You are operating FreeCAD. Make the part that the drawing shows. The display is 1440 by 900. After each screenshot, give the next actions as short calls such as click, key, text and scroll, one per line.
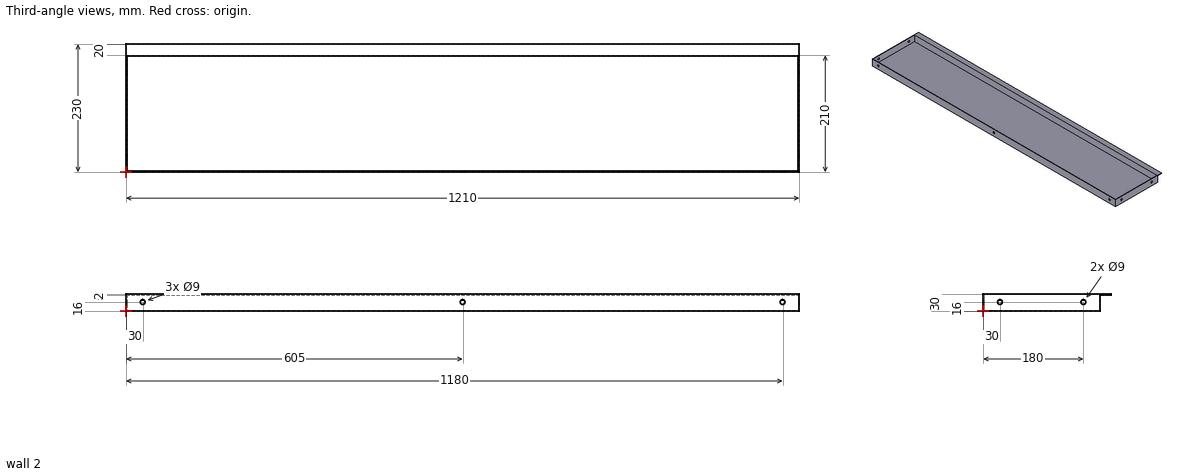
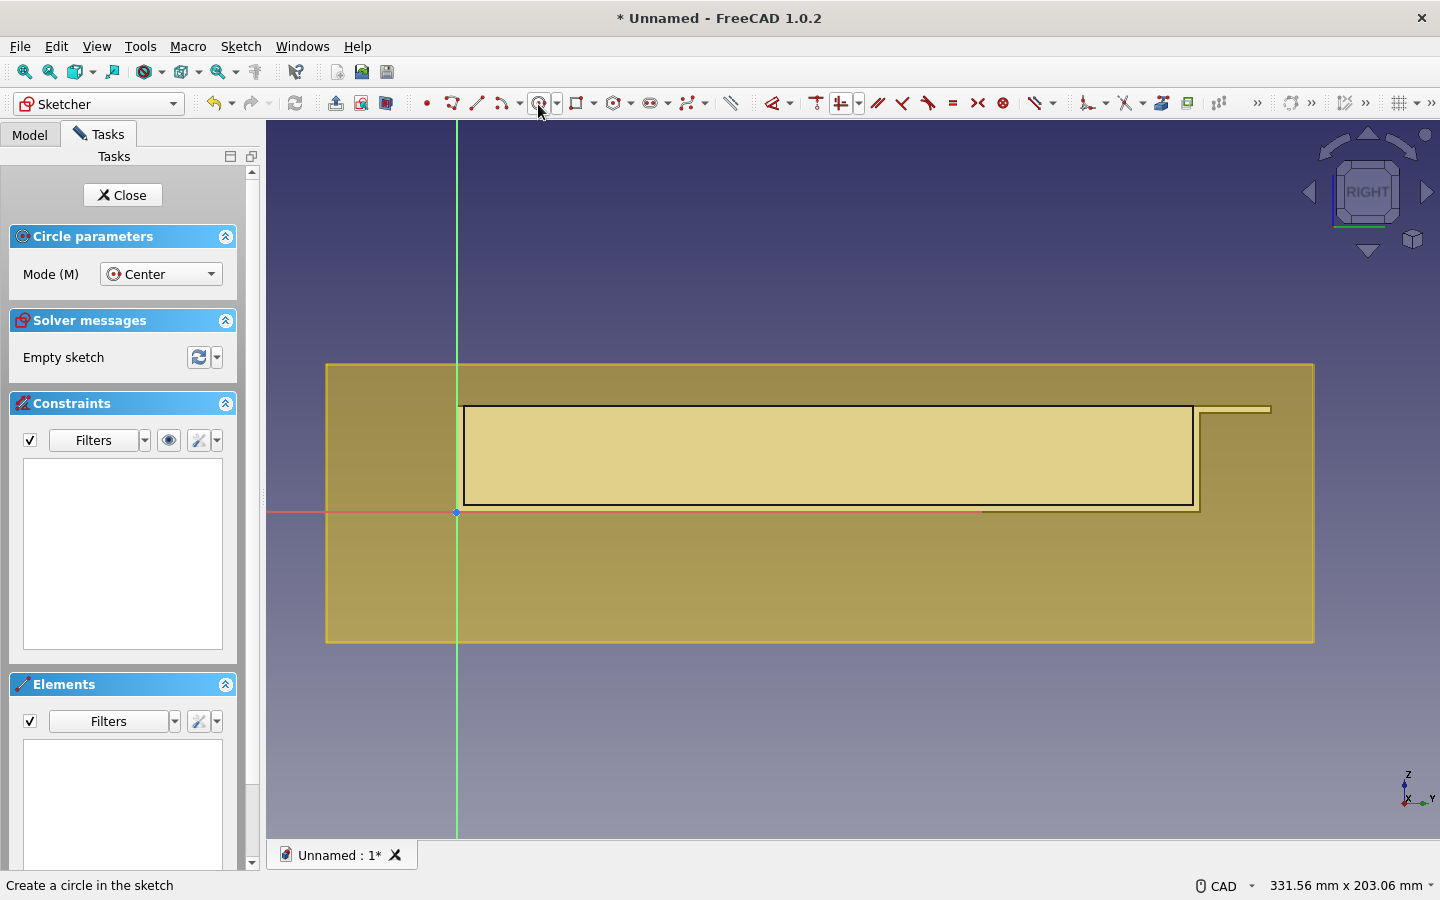
scroll(1094, 456, up, 2)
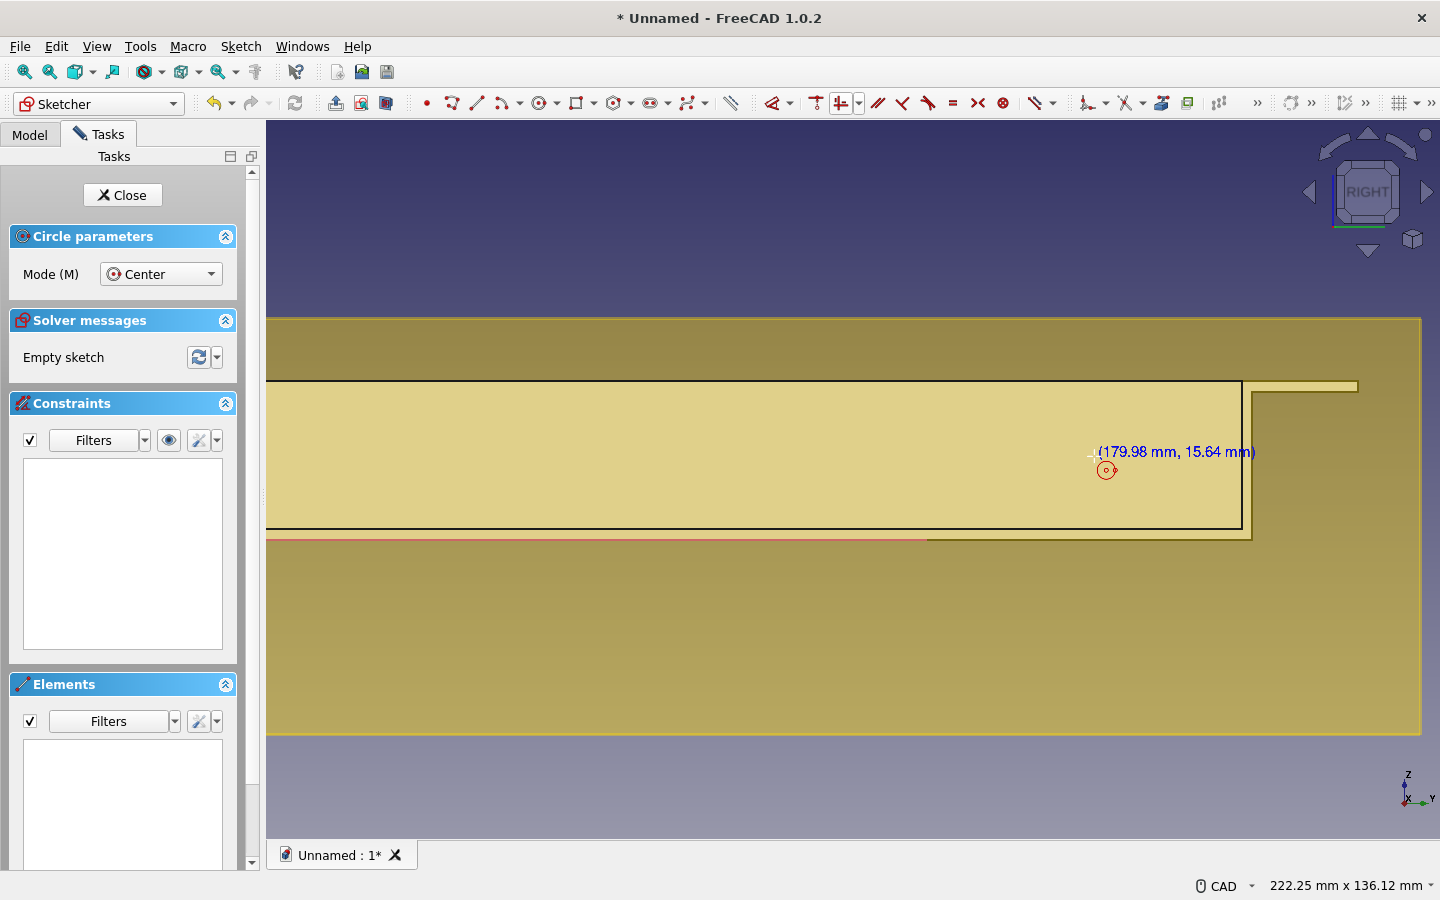
click(1094, 455)
click(1111, 439)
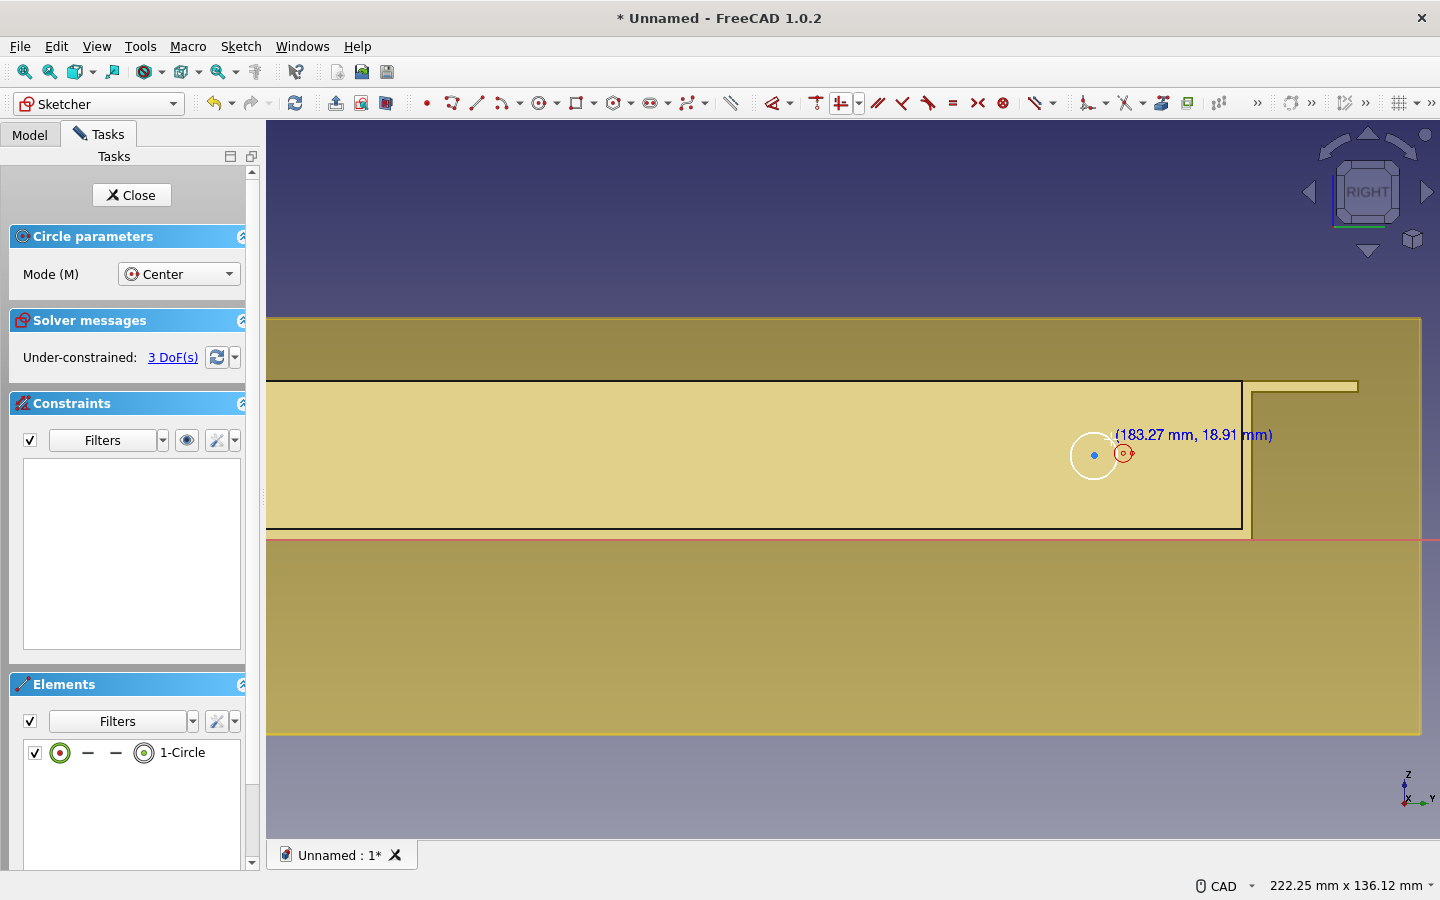
click(301, 455)
click(318, 439)
key(Escape)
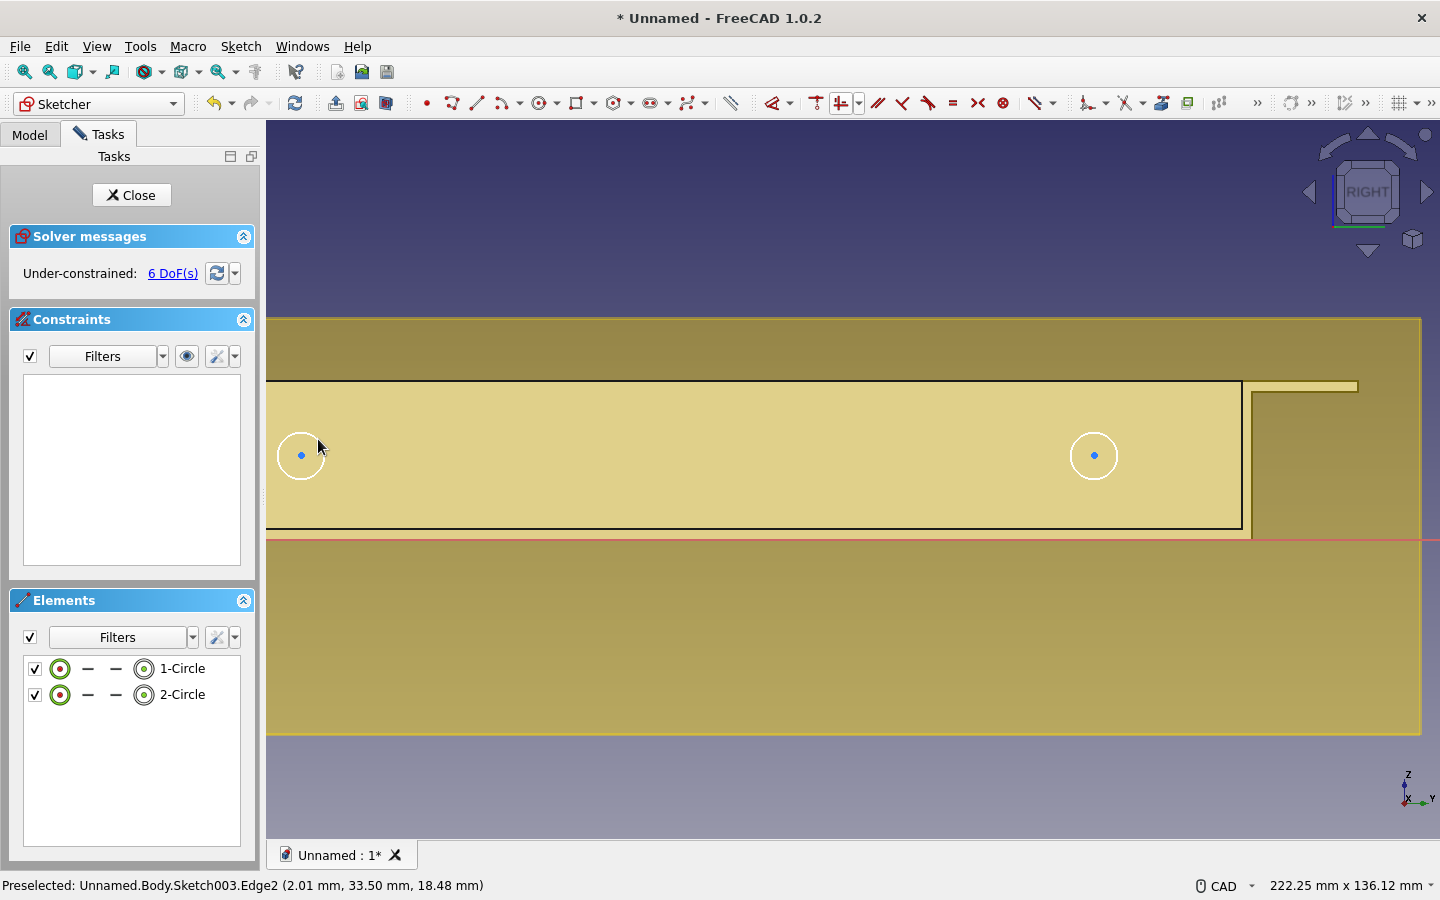
click(1110, 439)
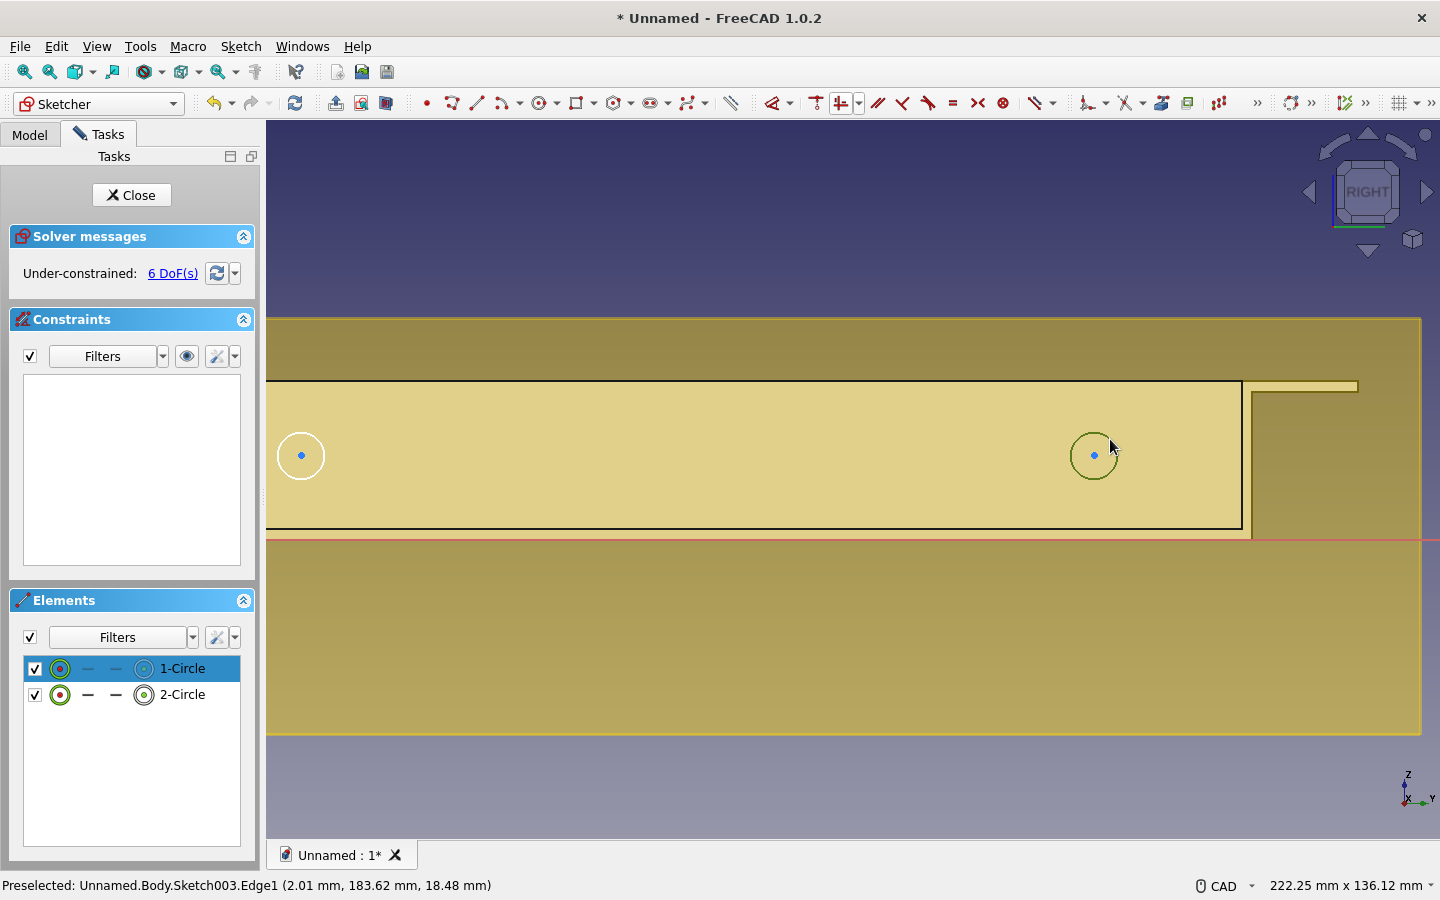
click(317, 439)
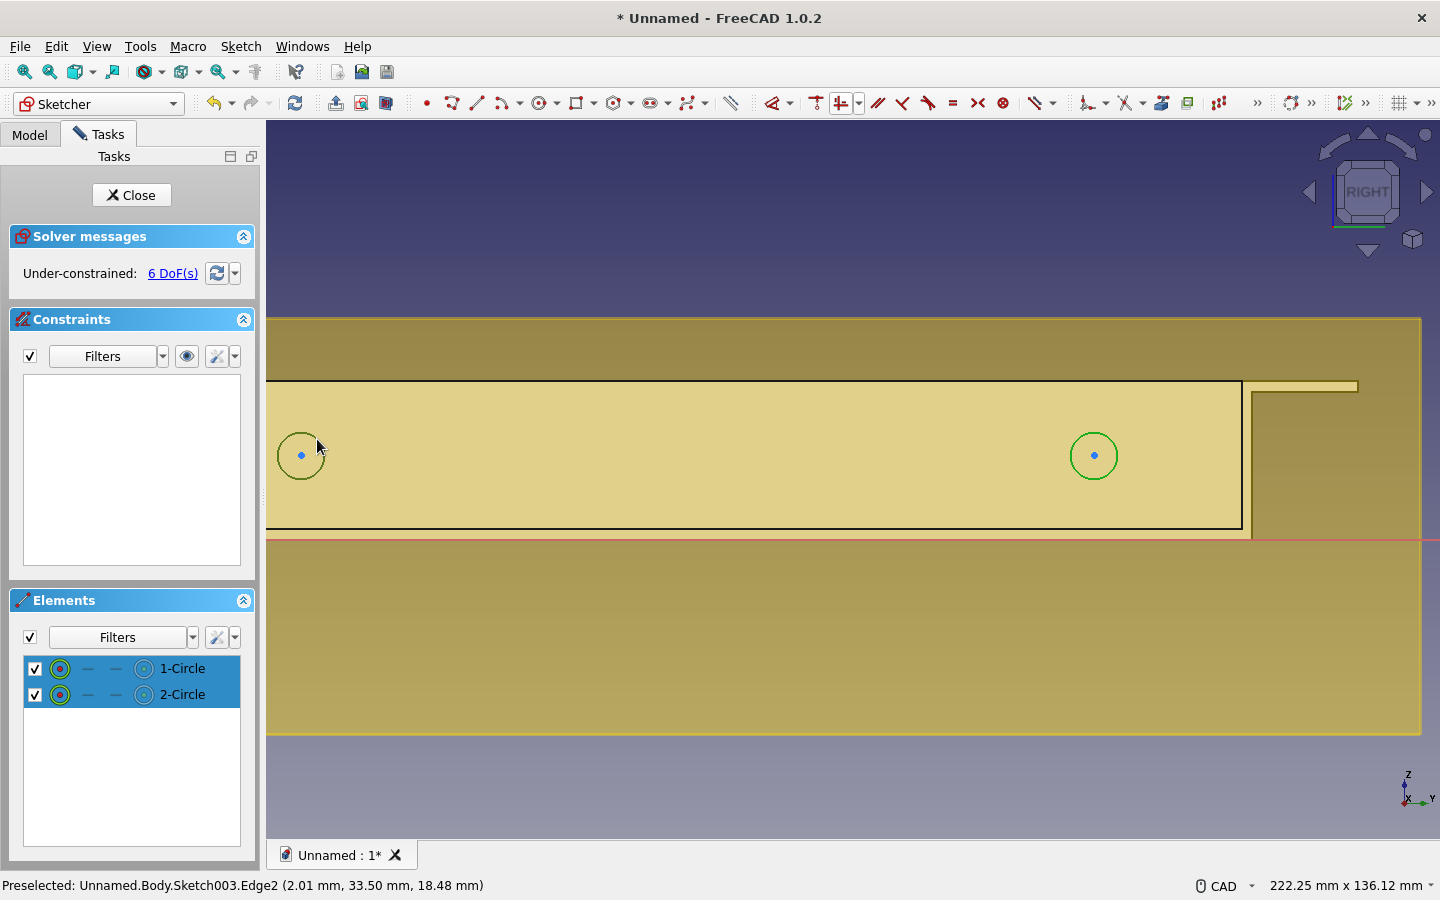
click(953, 104)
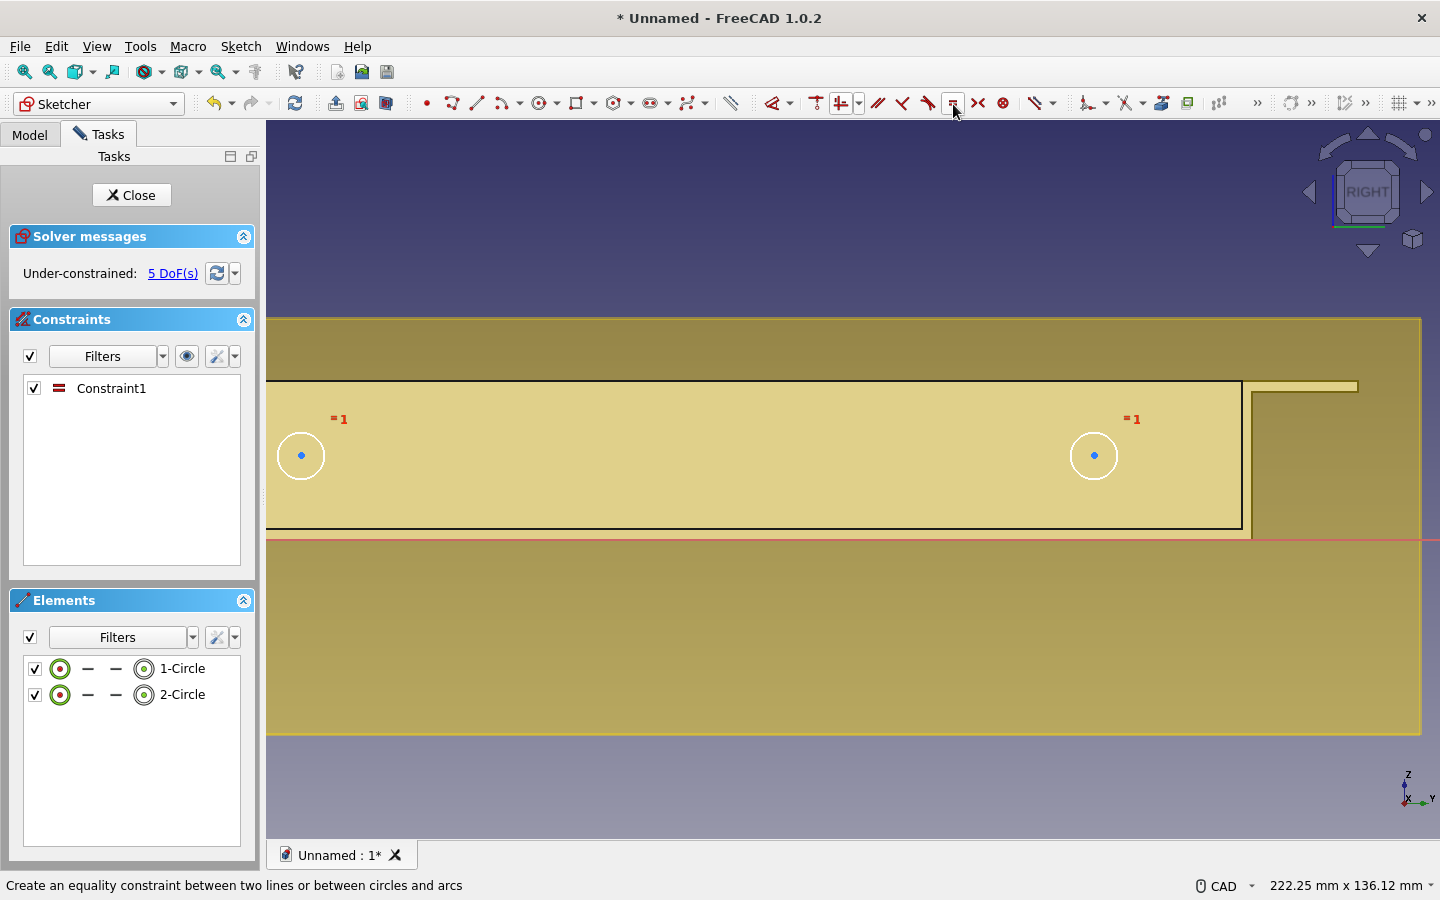
click(1094, 456)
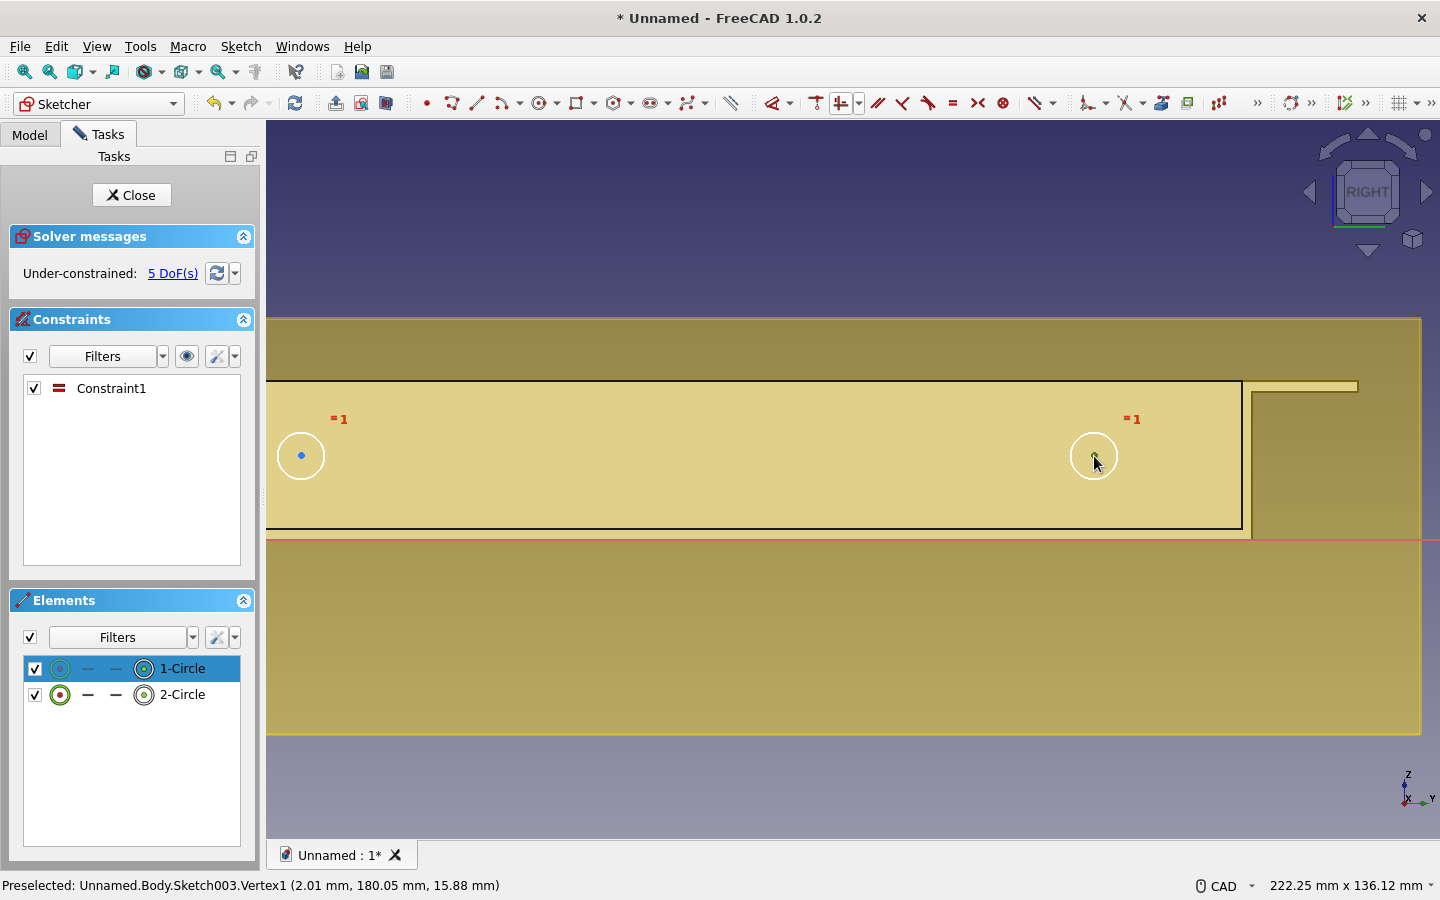
click(301, 456)